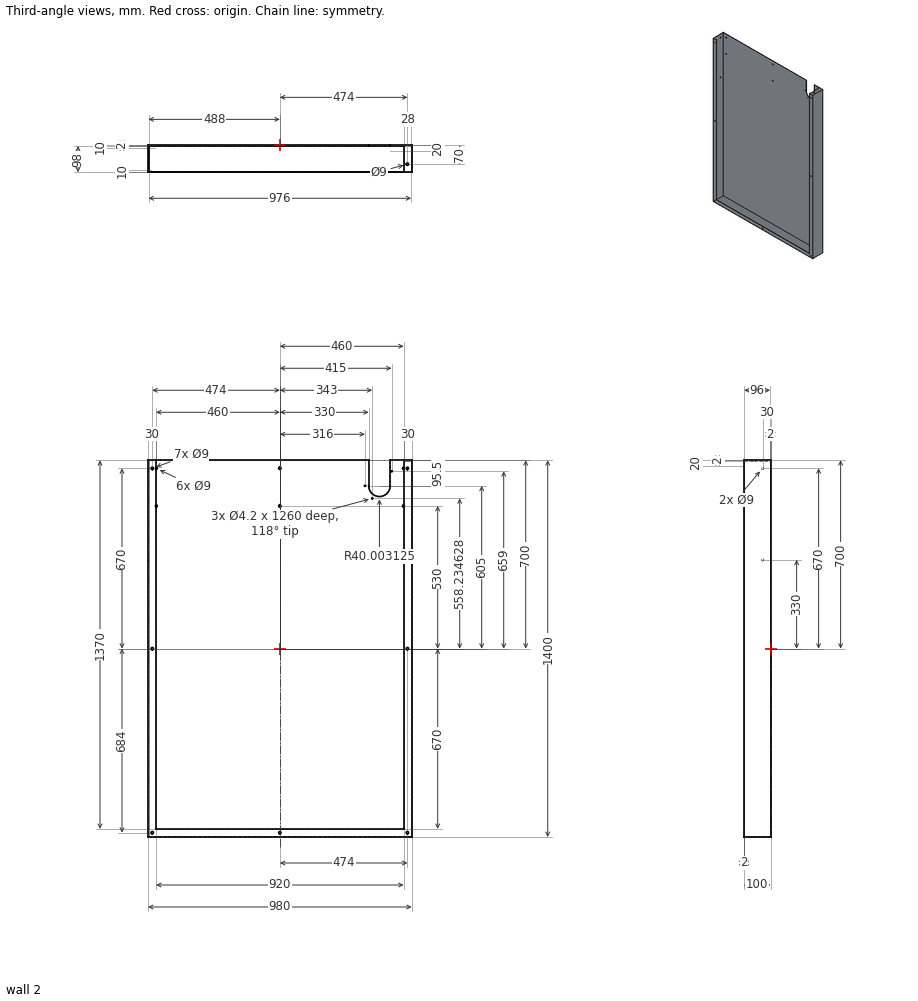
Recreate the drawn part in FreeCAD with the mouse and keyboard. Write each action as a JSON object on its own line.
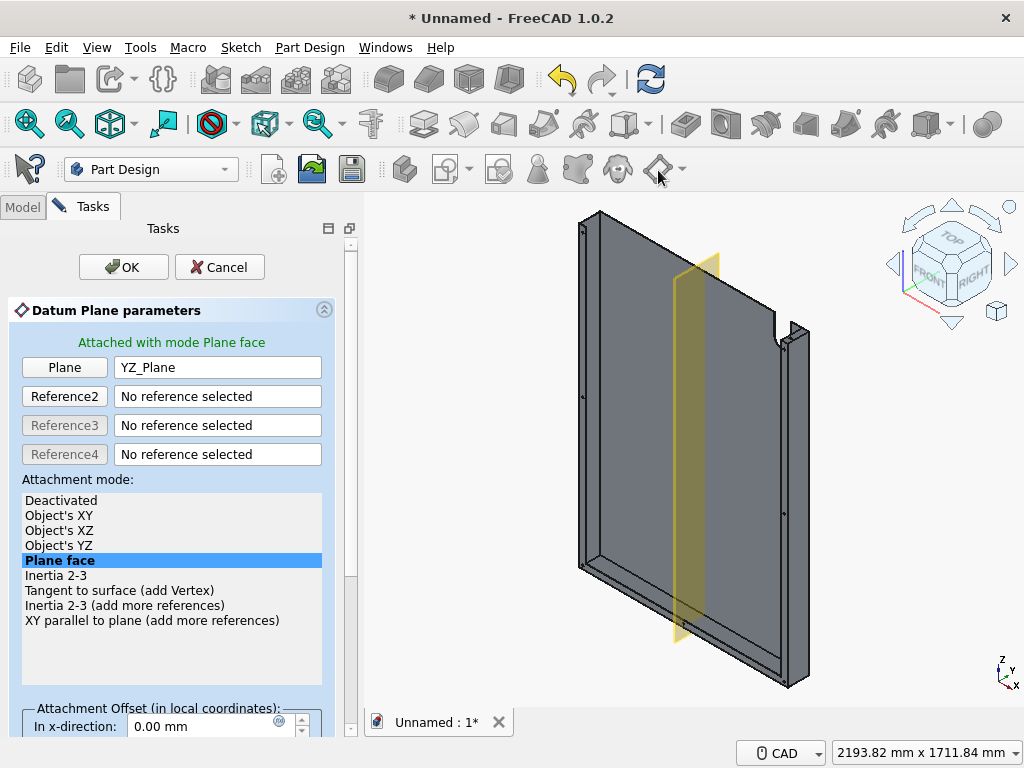
{"action": "scroll", "coordinate": [351, 487], "scroll_direction": "down", "scroll_amount": 3}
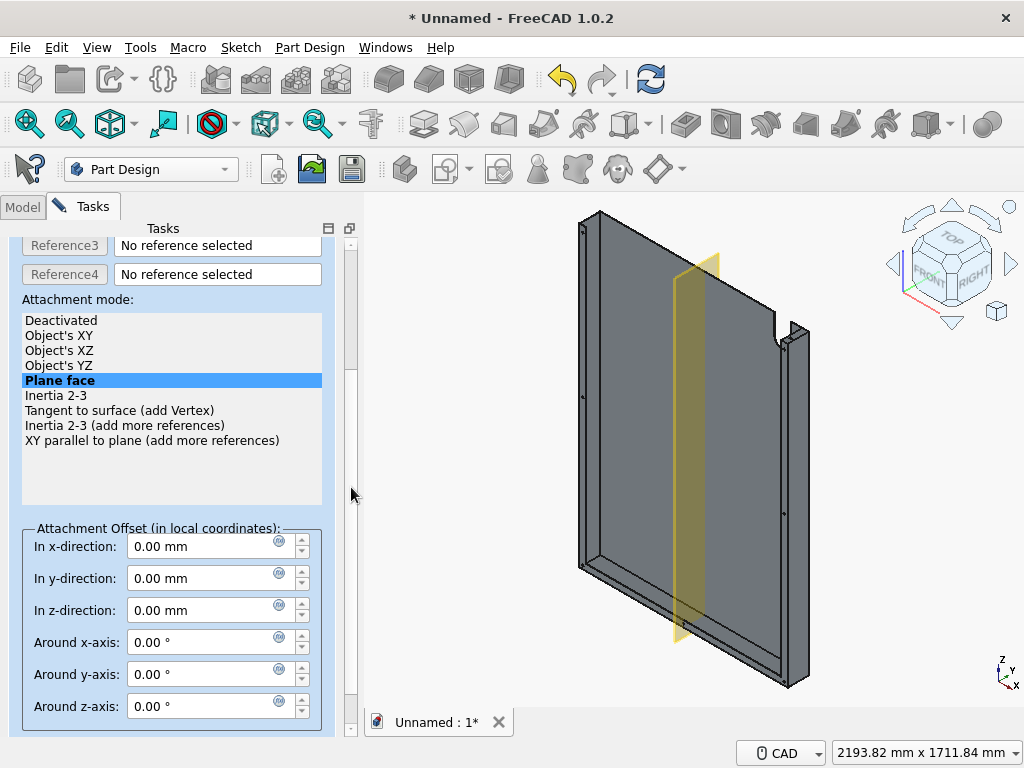
{"action": "triple_click", "coordinate": [210, 610]}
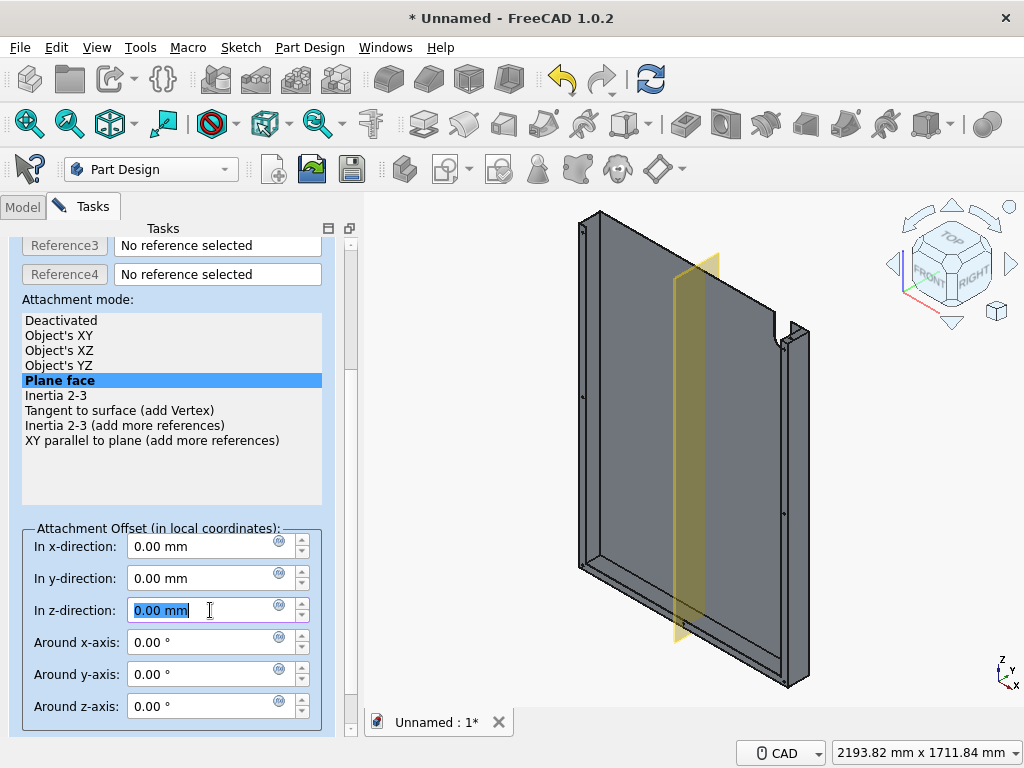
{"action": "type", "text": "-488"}
{"action": "key", "text": "Tab"}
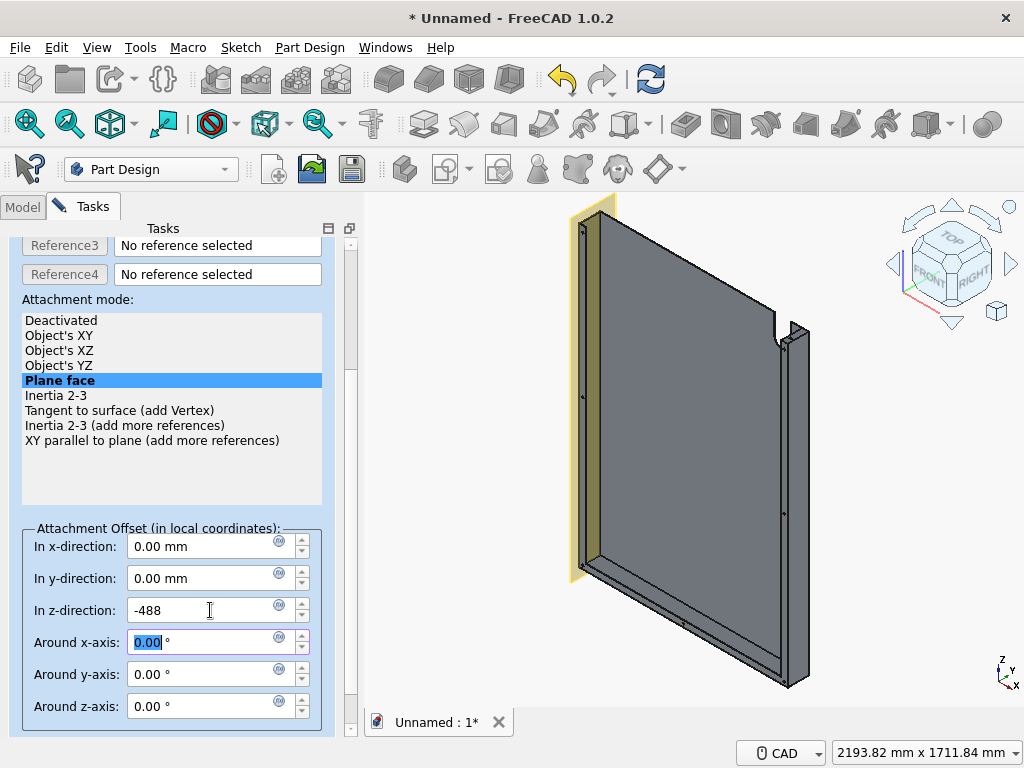
{"action": "scroll", "coordinate": [351, 487], "scroll_direction": "up", "scroll_amount": 4}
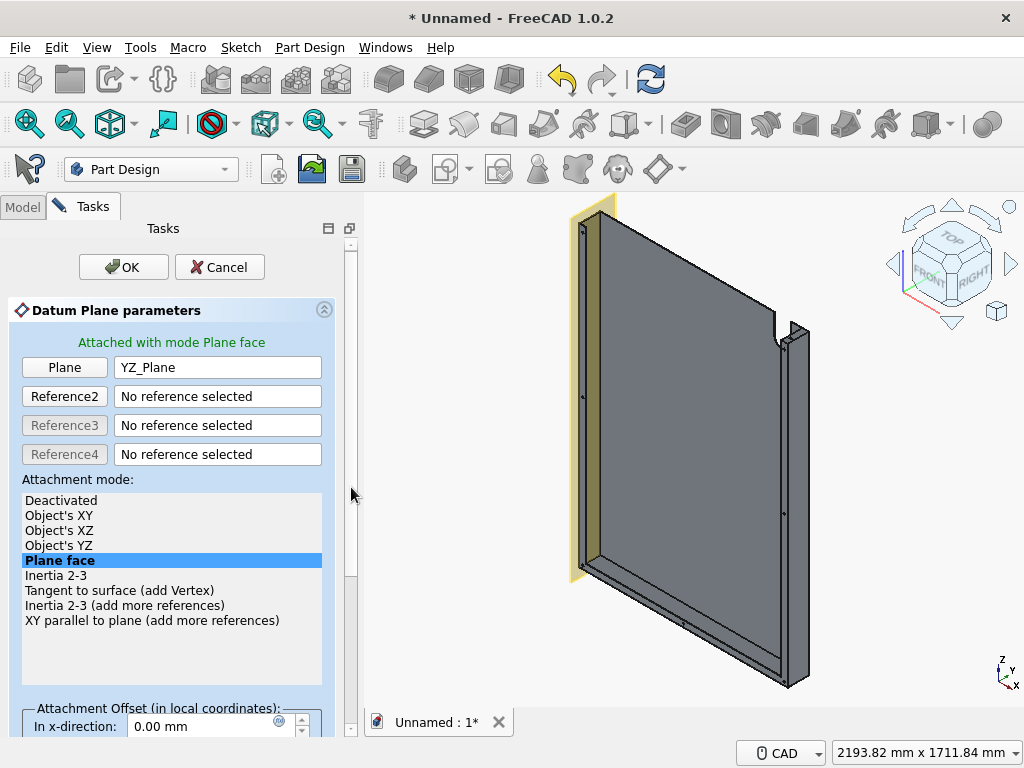
{"action": "left_click", "coordinate": [124, 267]}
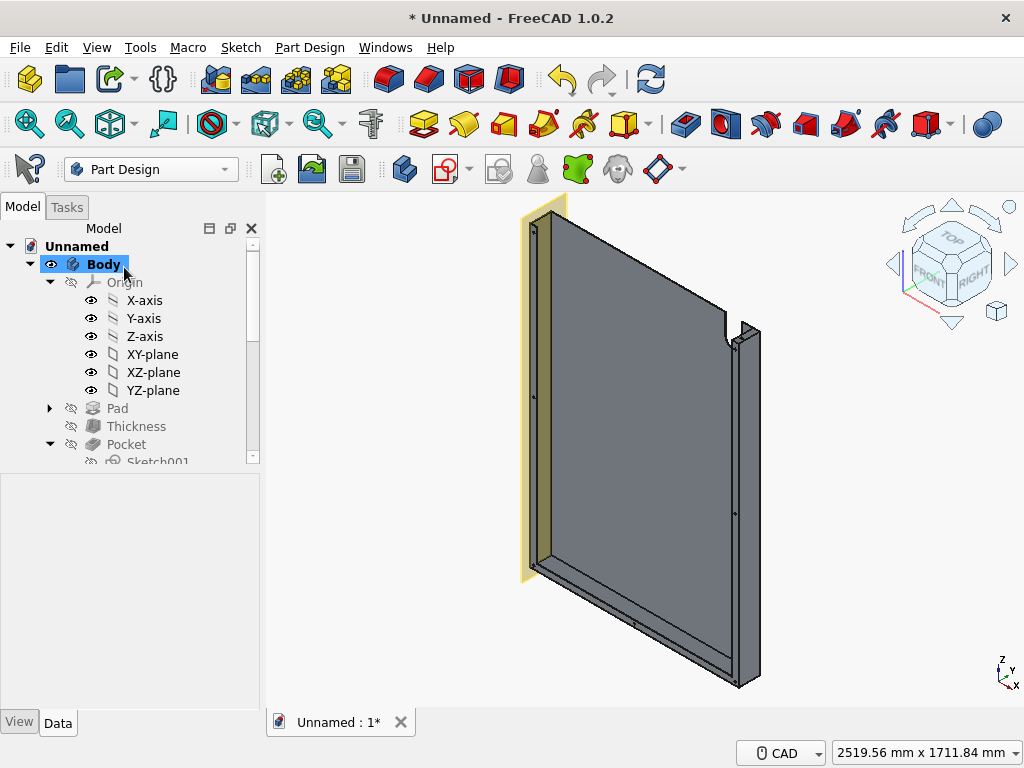
{"action": "scroll", "coordinate": [100, 350], "scroll_direction": "down", "scroll_amount": 3}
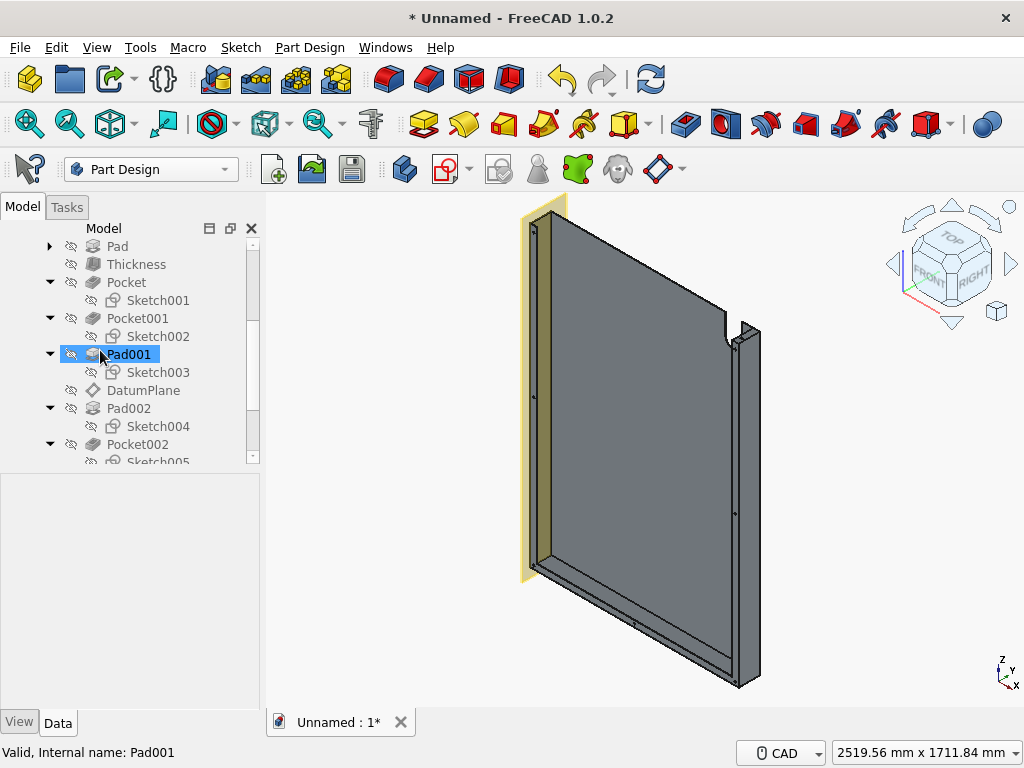
{"action": "scroll", "coordinate": [140, 350], "scroll_direction": "up", "scroll_amount": 15}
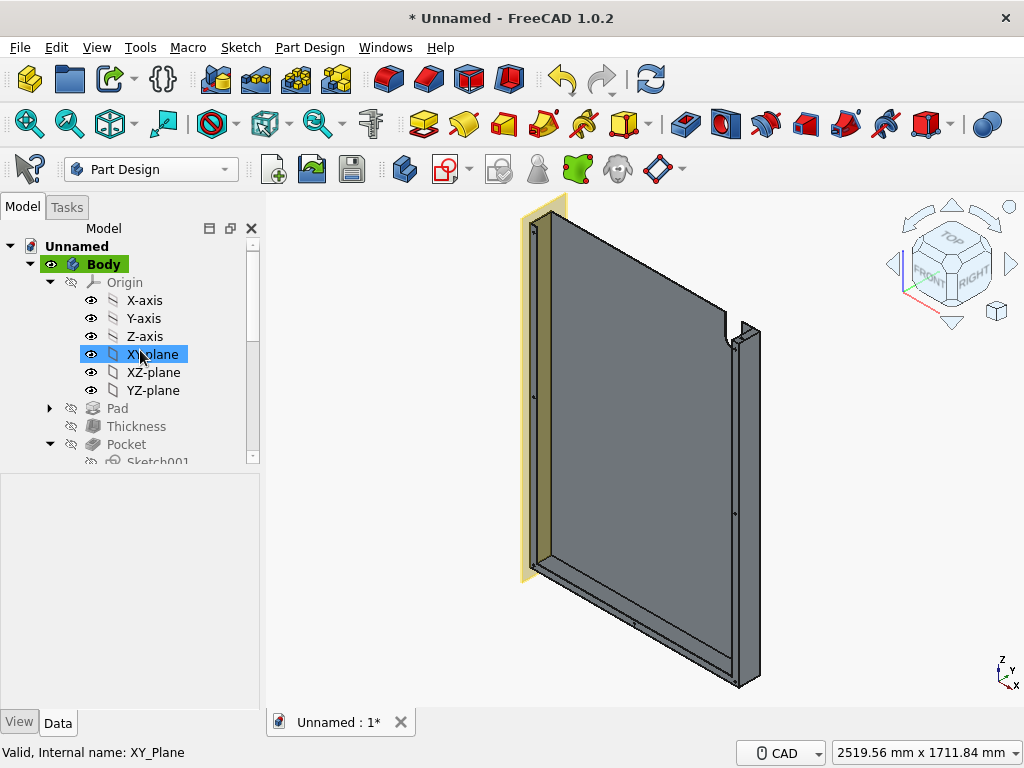
{"action": "scroll", "coordinate": [100, 350], "scroll_direction": "down", "scroll_amount": 6}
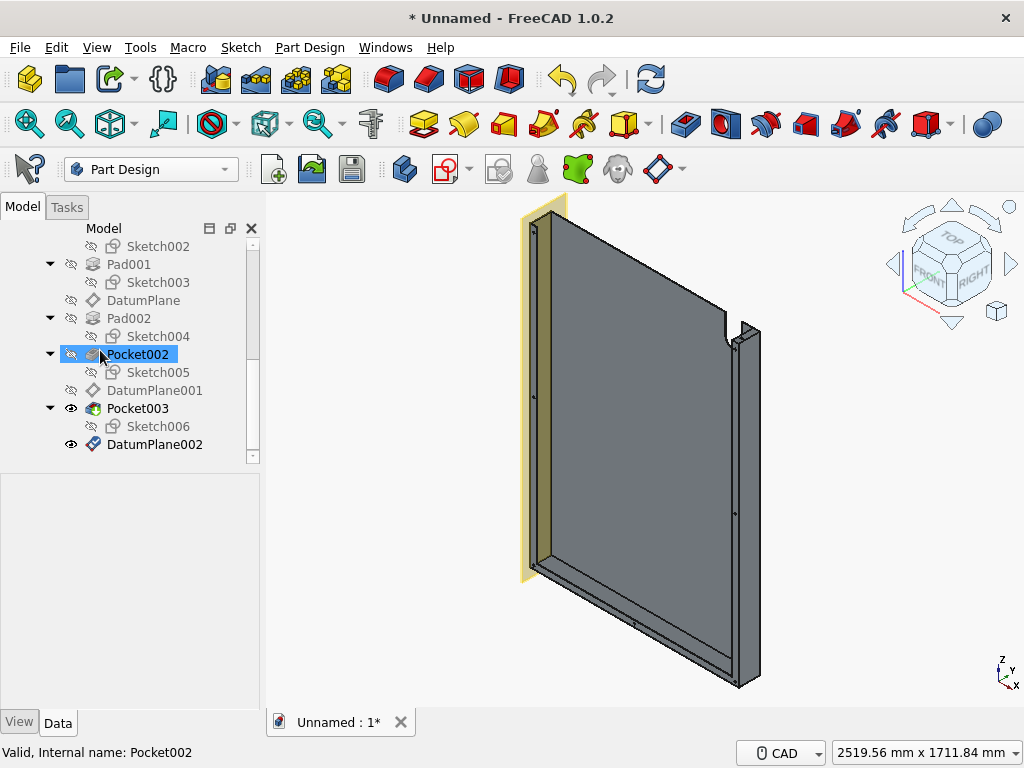
{"action": "left_click", "coordinate": [116, 444]}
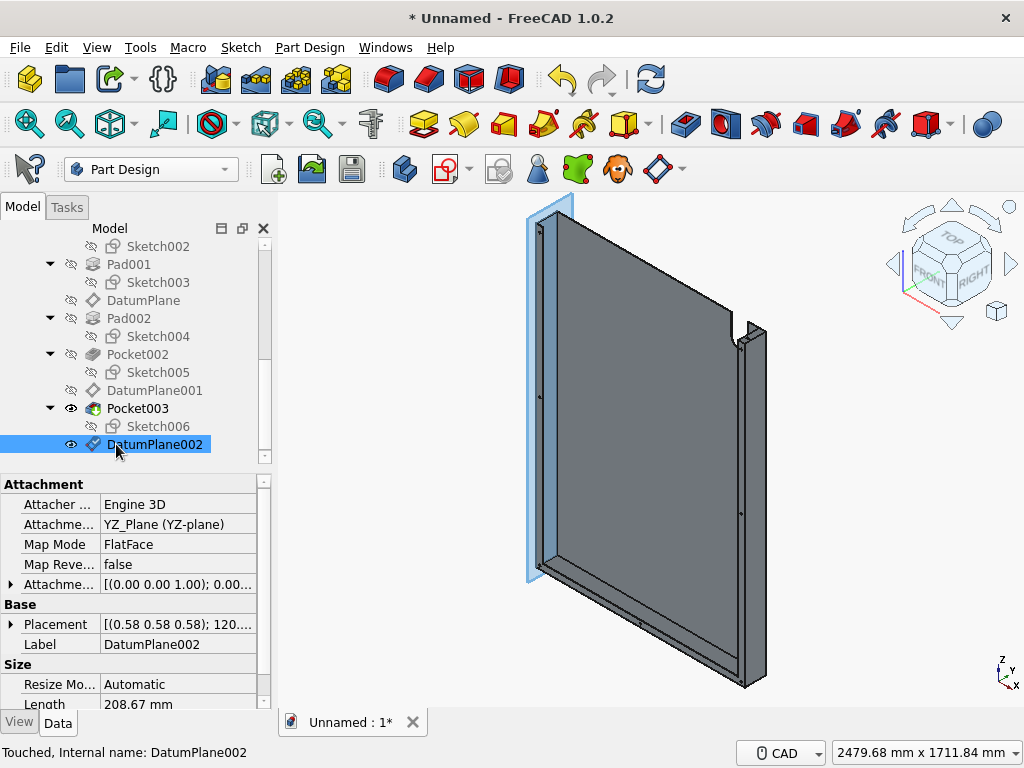
{"action": "left_click", "coordinate": [446, 170]}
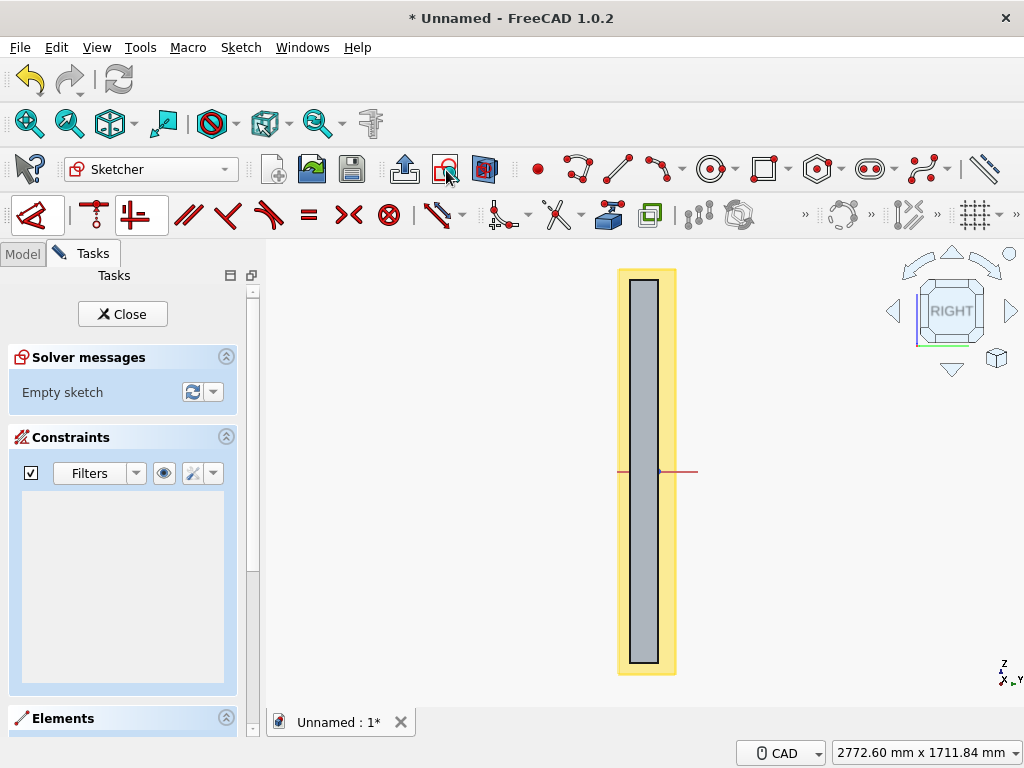
{"action": "left_click", "coordinate": [486, 170]}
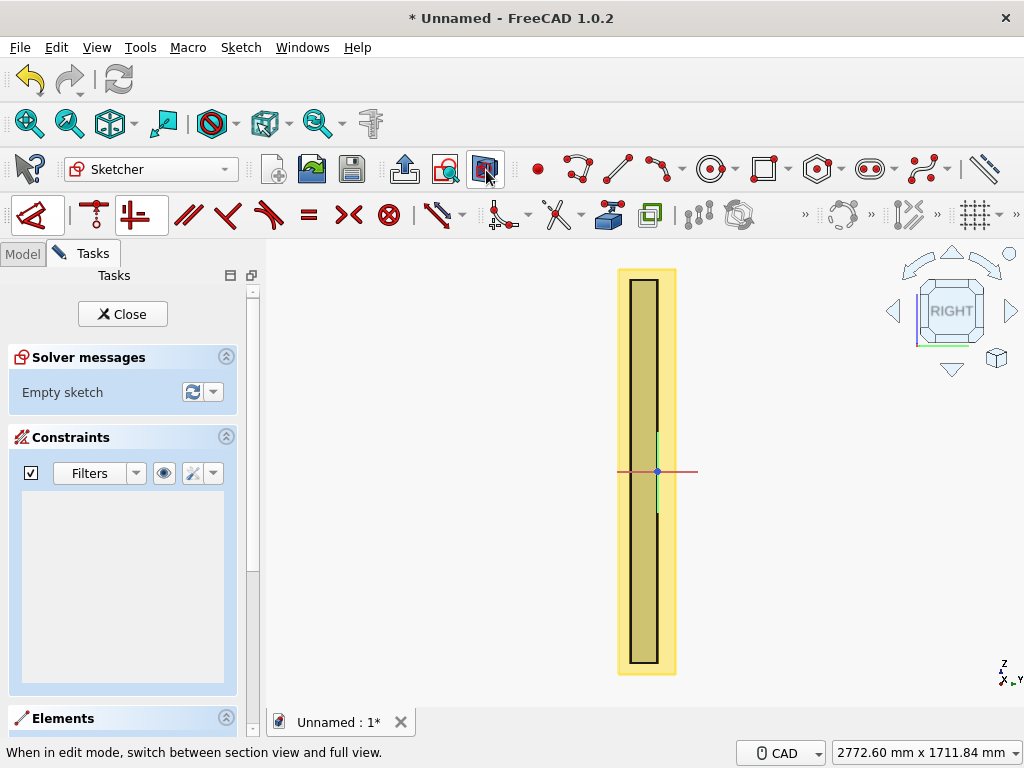
{"action": "scroll", "coordinate": [808, 267], "scroll_direction": "up", "scroll_amount": 2}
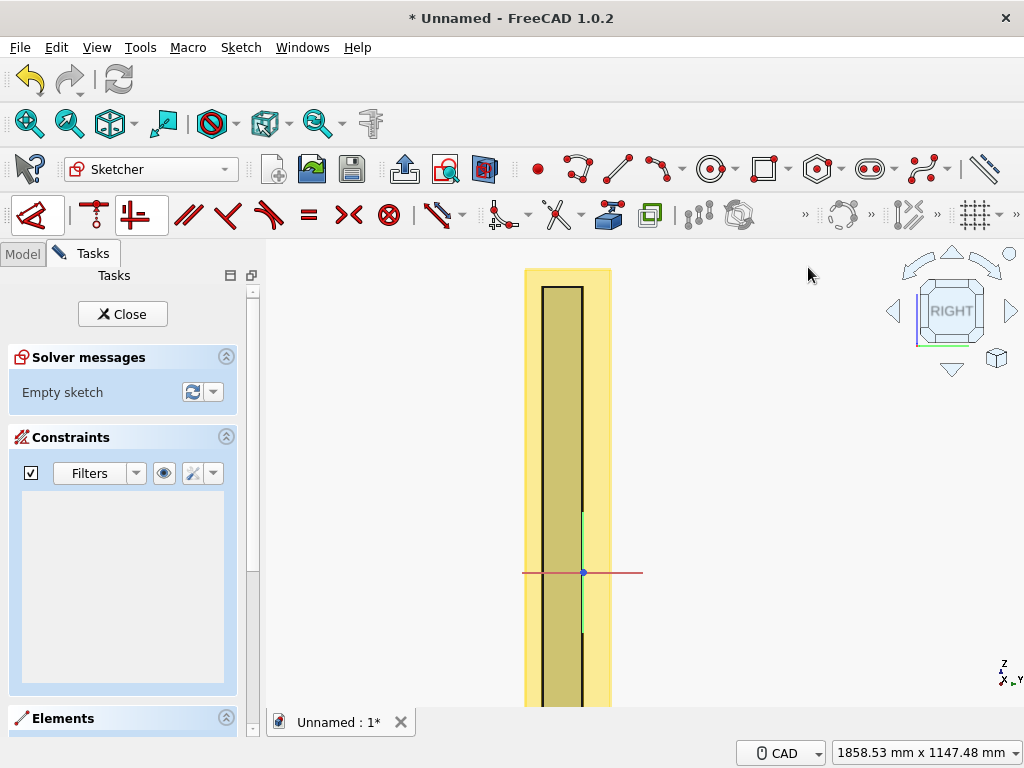
{"action": "left_click", "coordinate": [712, 170]}